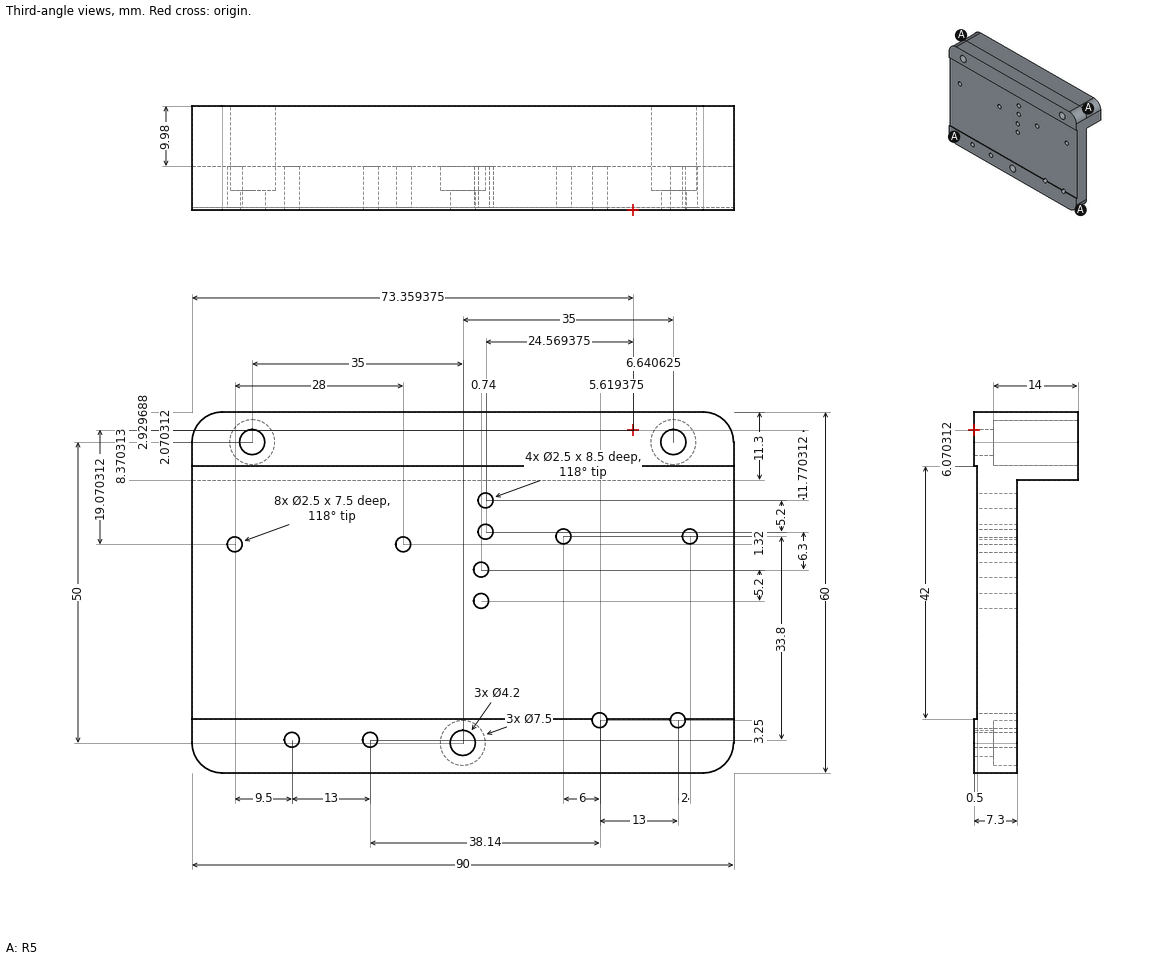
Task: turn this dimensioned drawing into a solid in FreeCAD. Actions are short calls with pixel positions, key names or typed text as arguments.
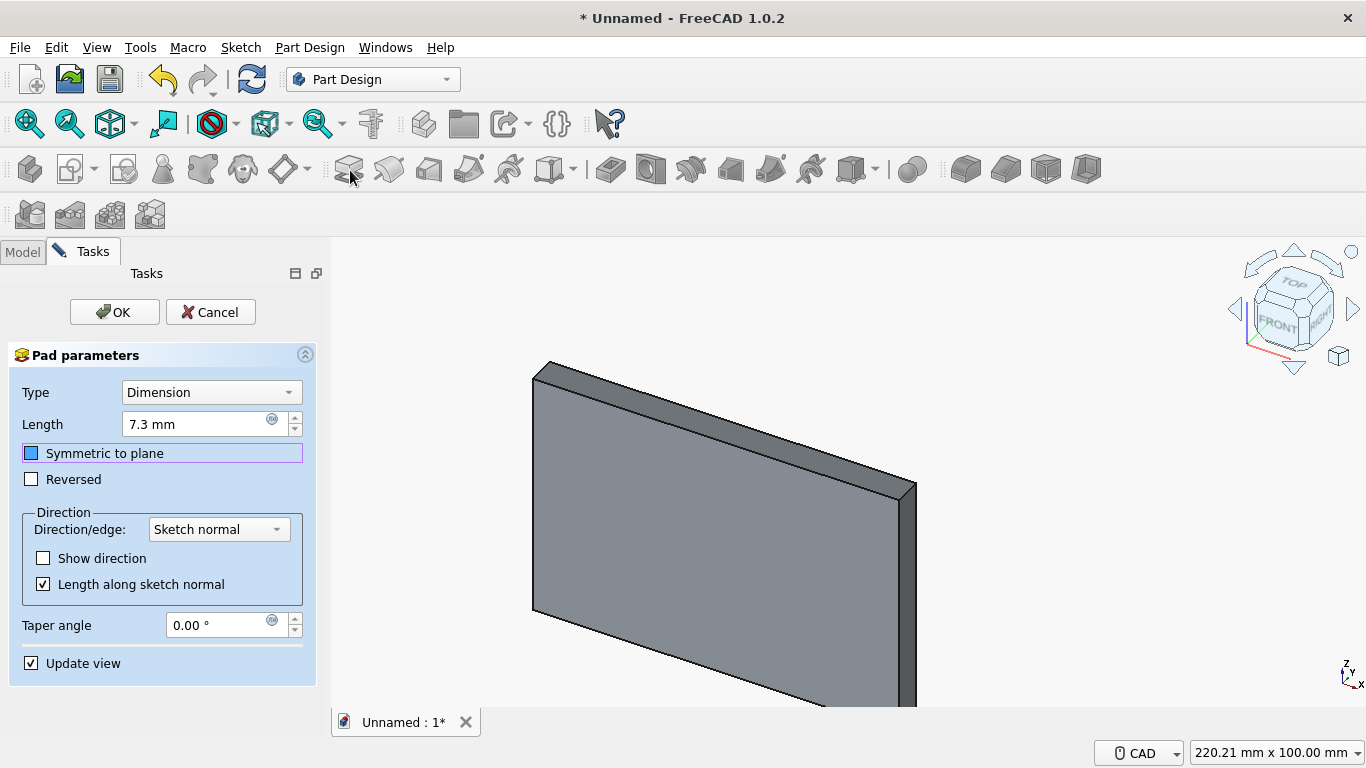
click(30, 479)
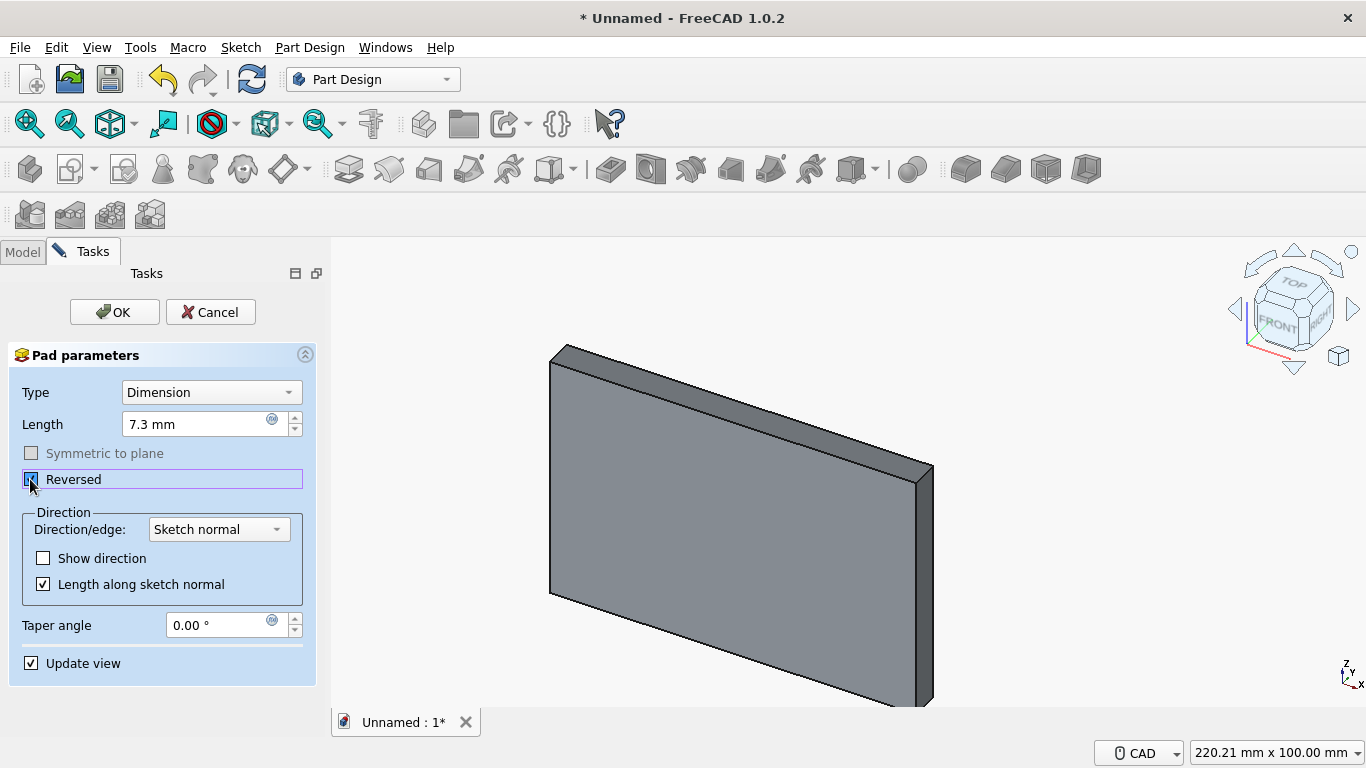
click(115, 312)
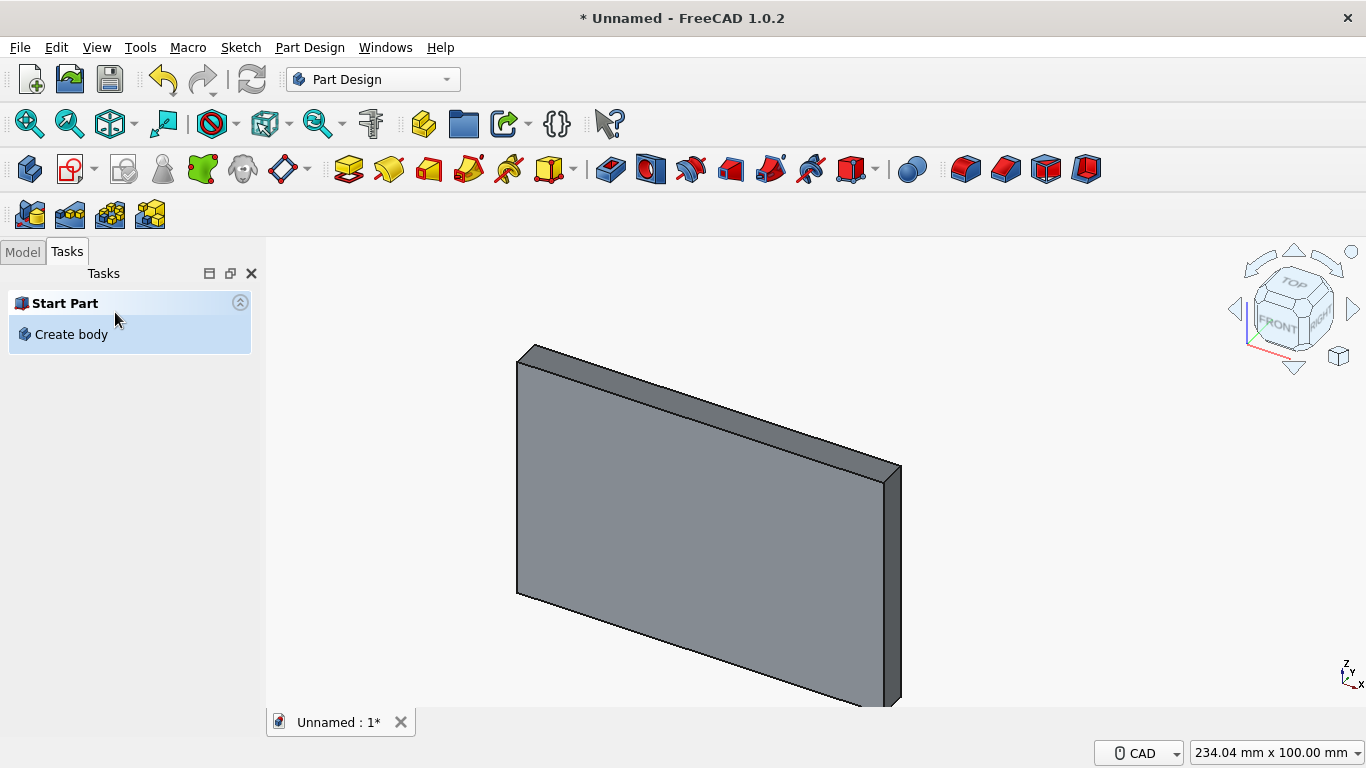
click(30, 124)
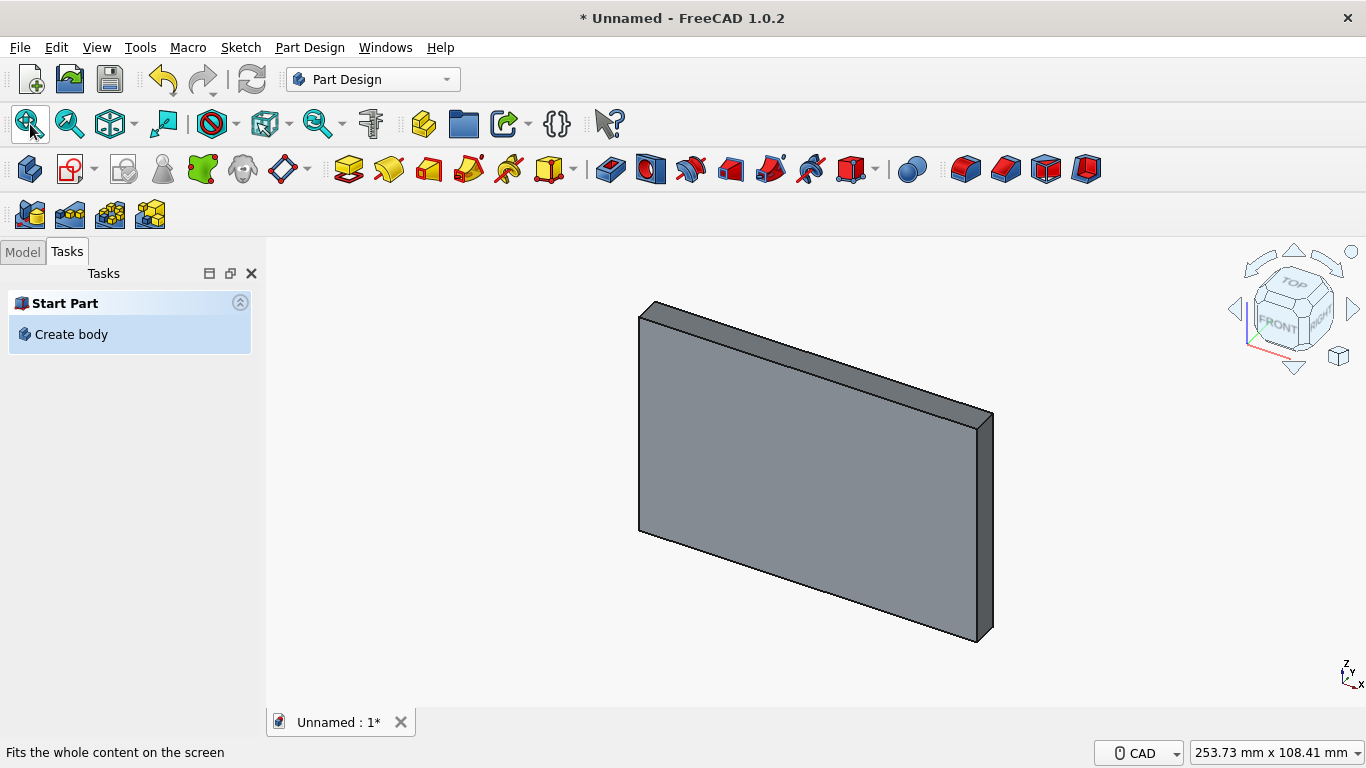
key(4)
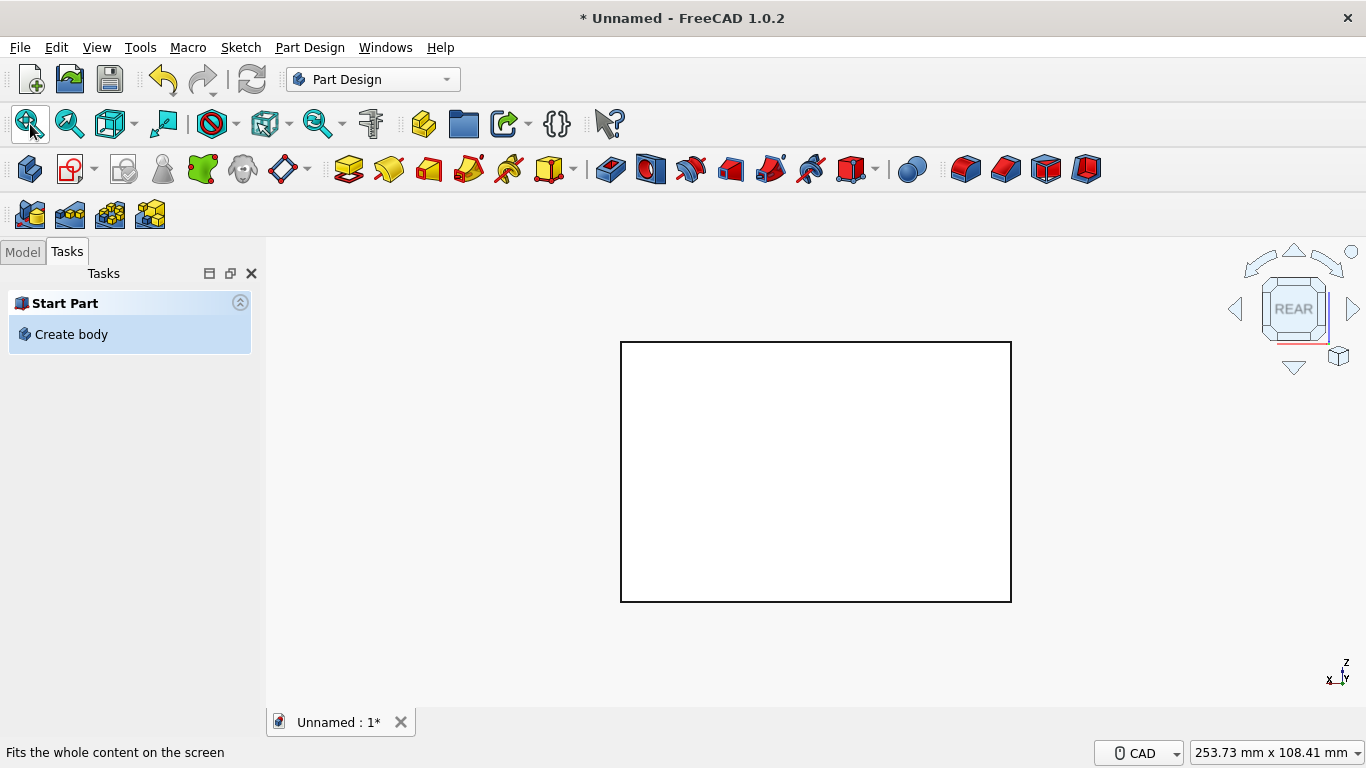
click(760, 471)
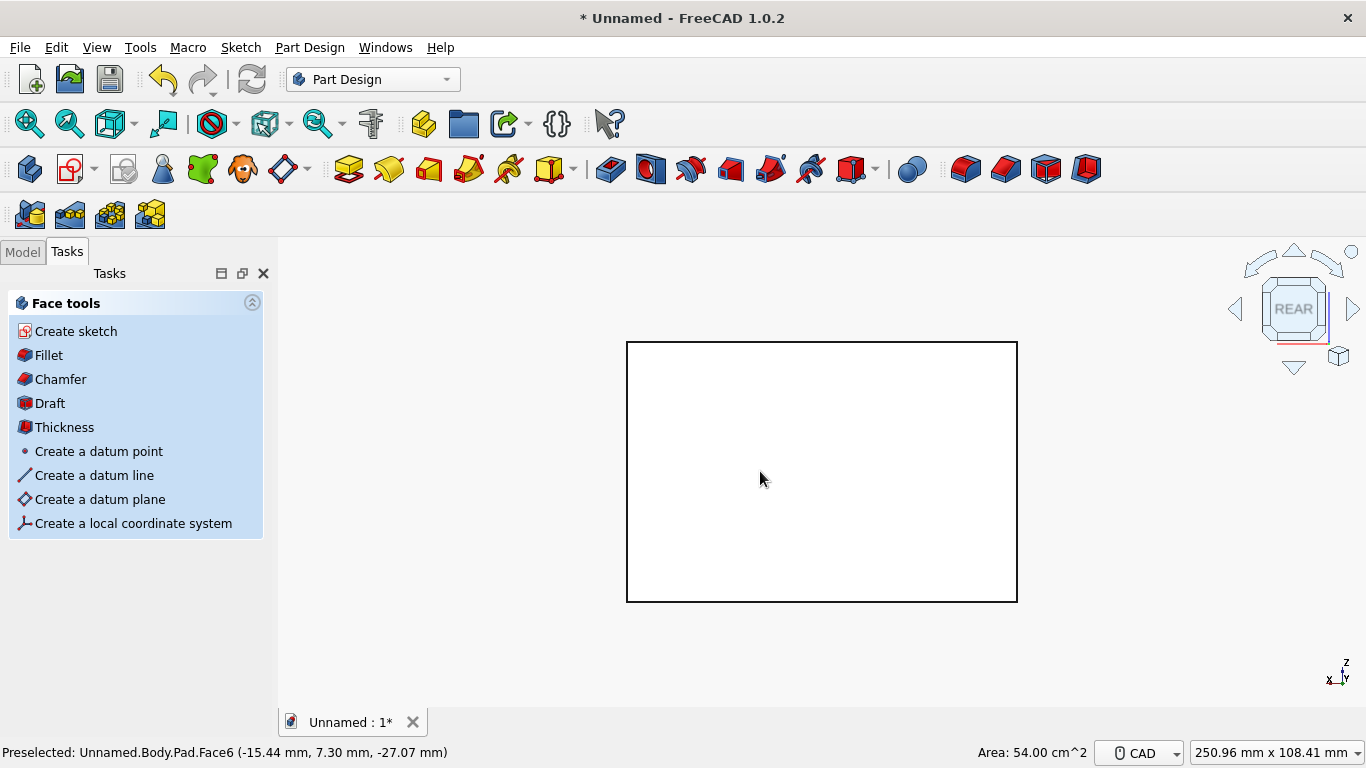
click(70, 170)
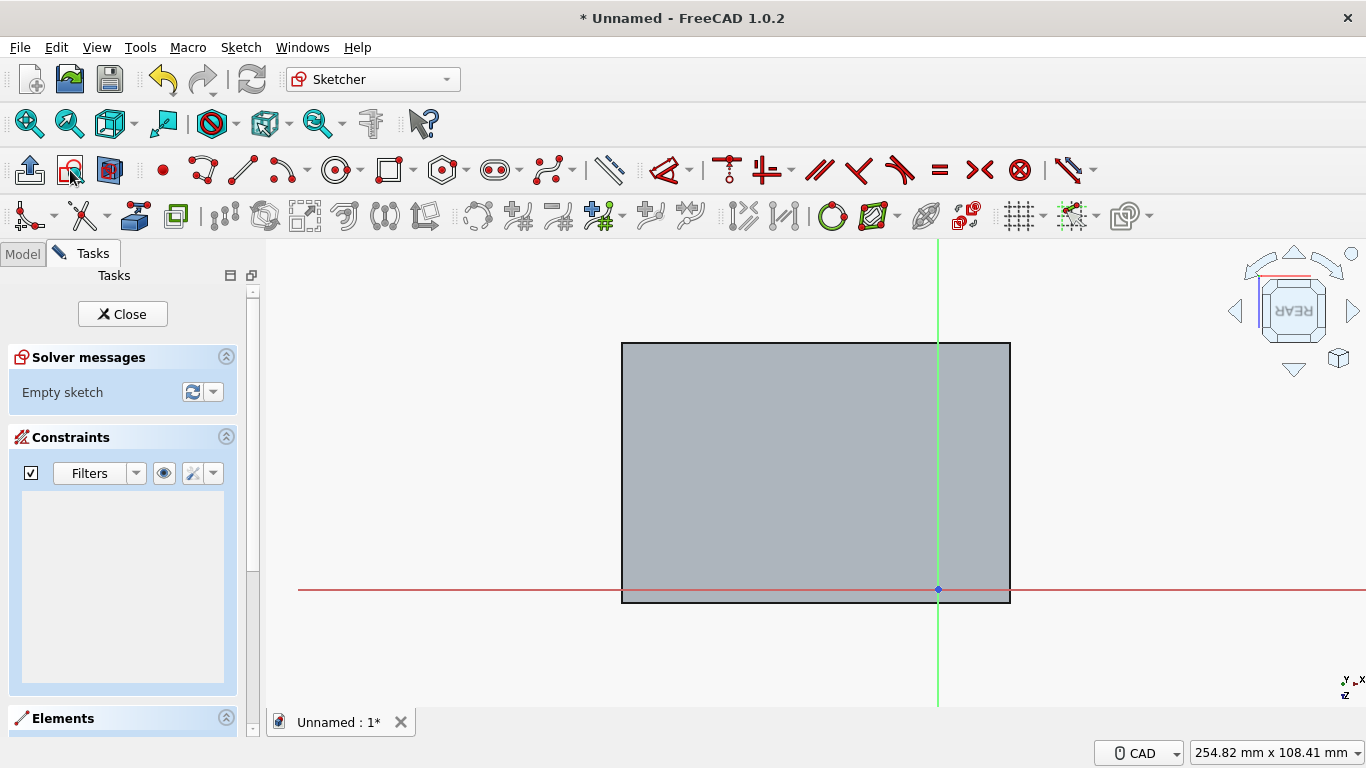
scroll(955, 679, up, 2)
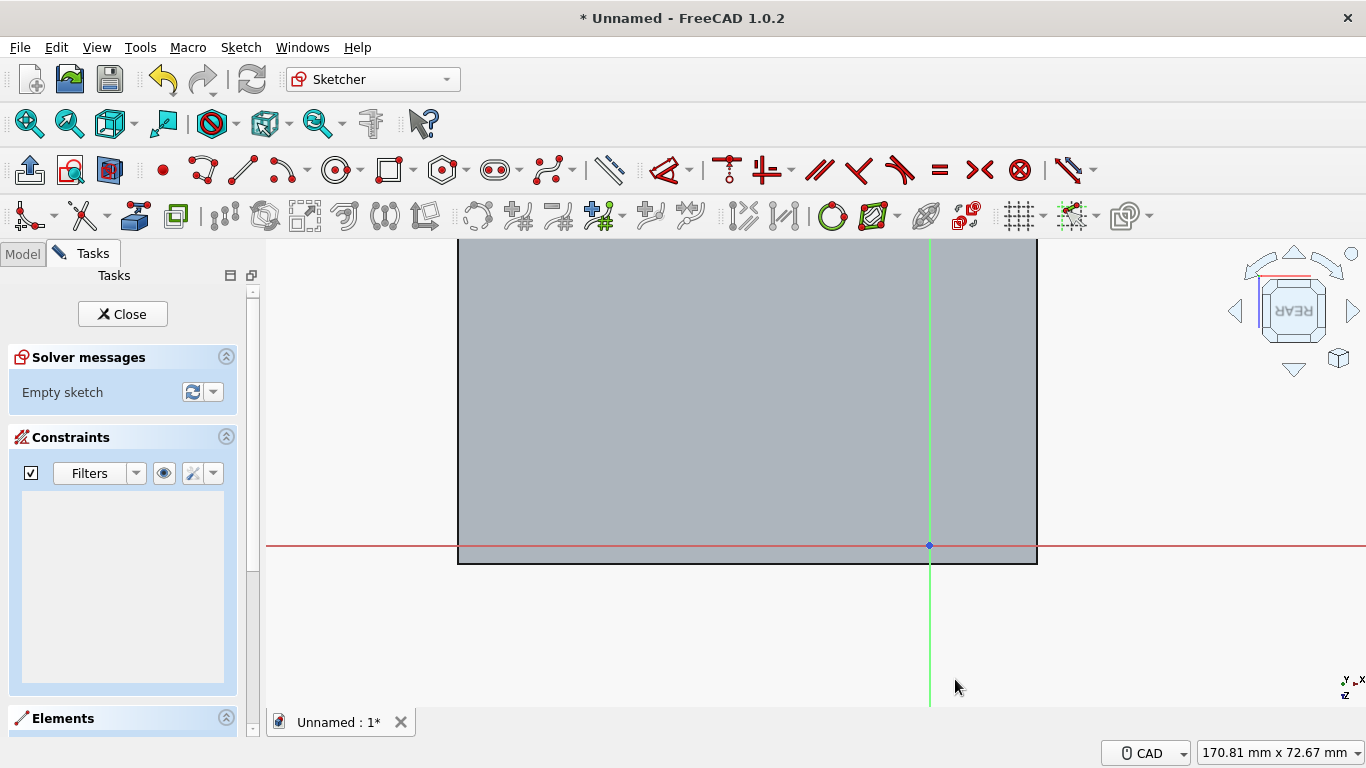
click(390, 170)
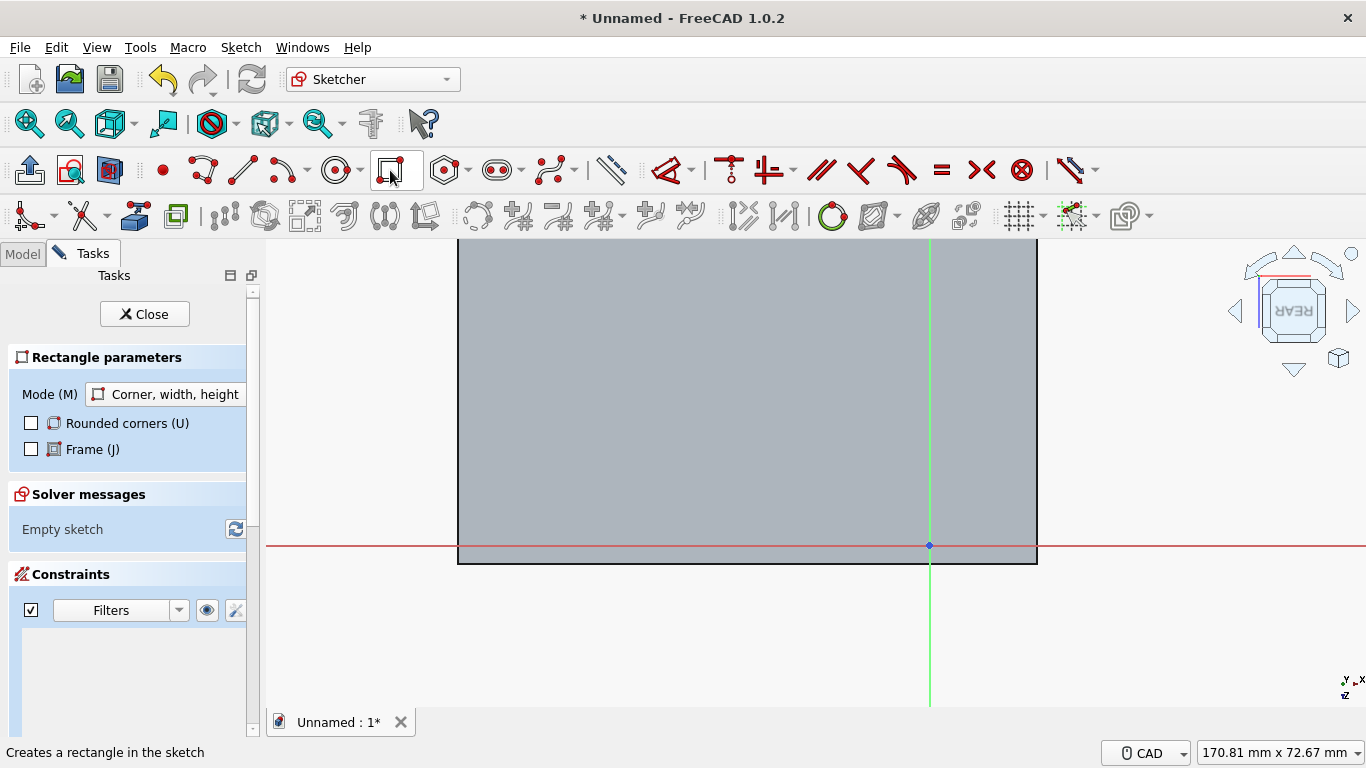
click(458, 492)
move(1037, 564)